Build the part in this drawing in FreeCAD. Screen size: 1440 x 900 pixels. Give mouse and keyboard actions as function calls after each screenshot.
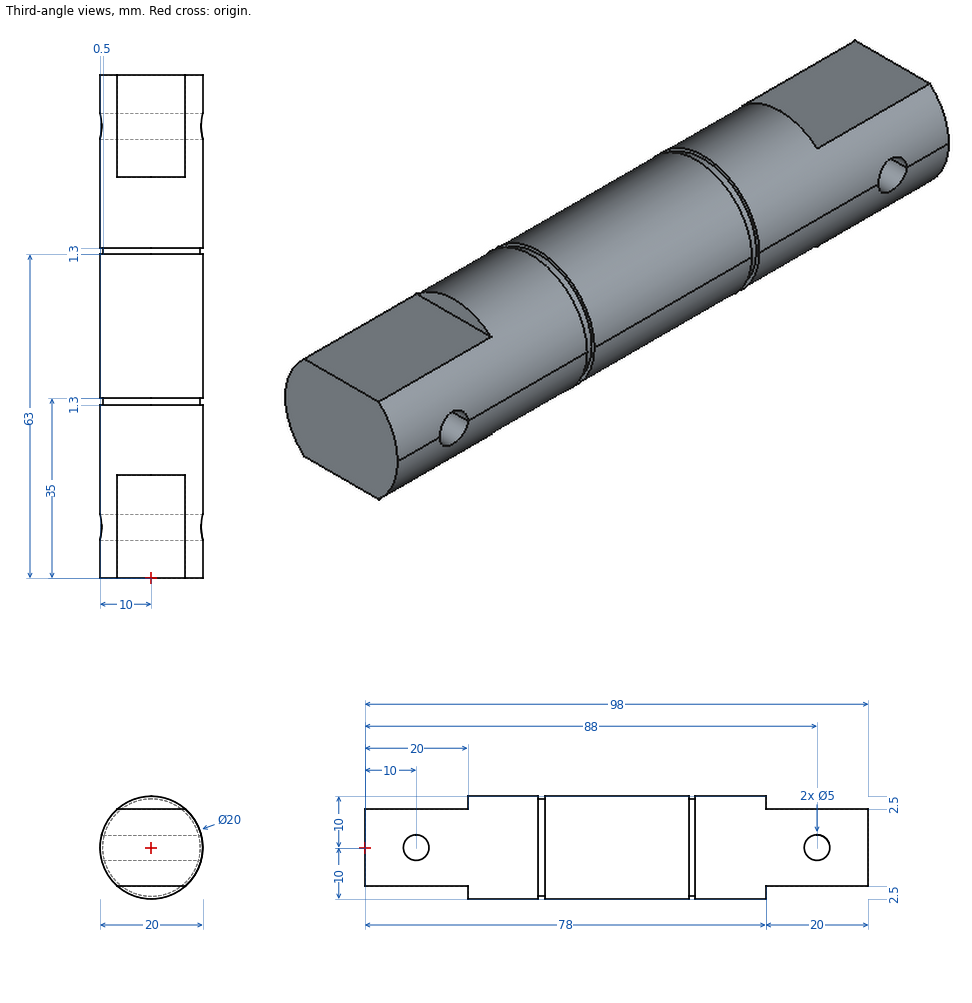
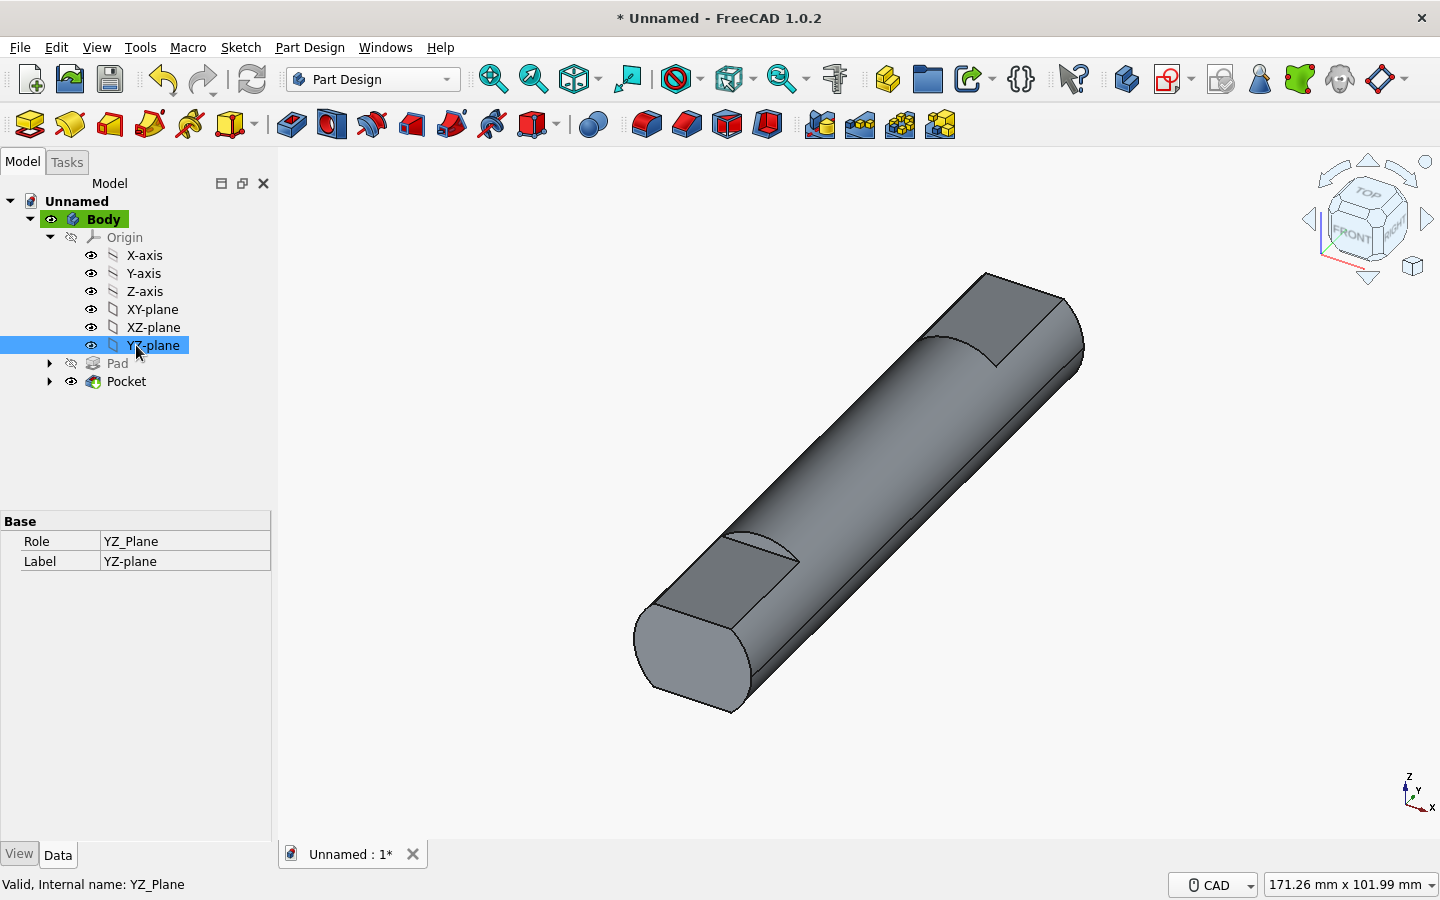
click(1380, 80)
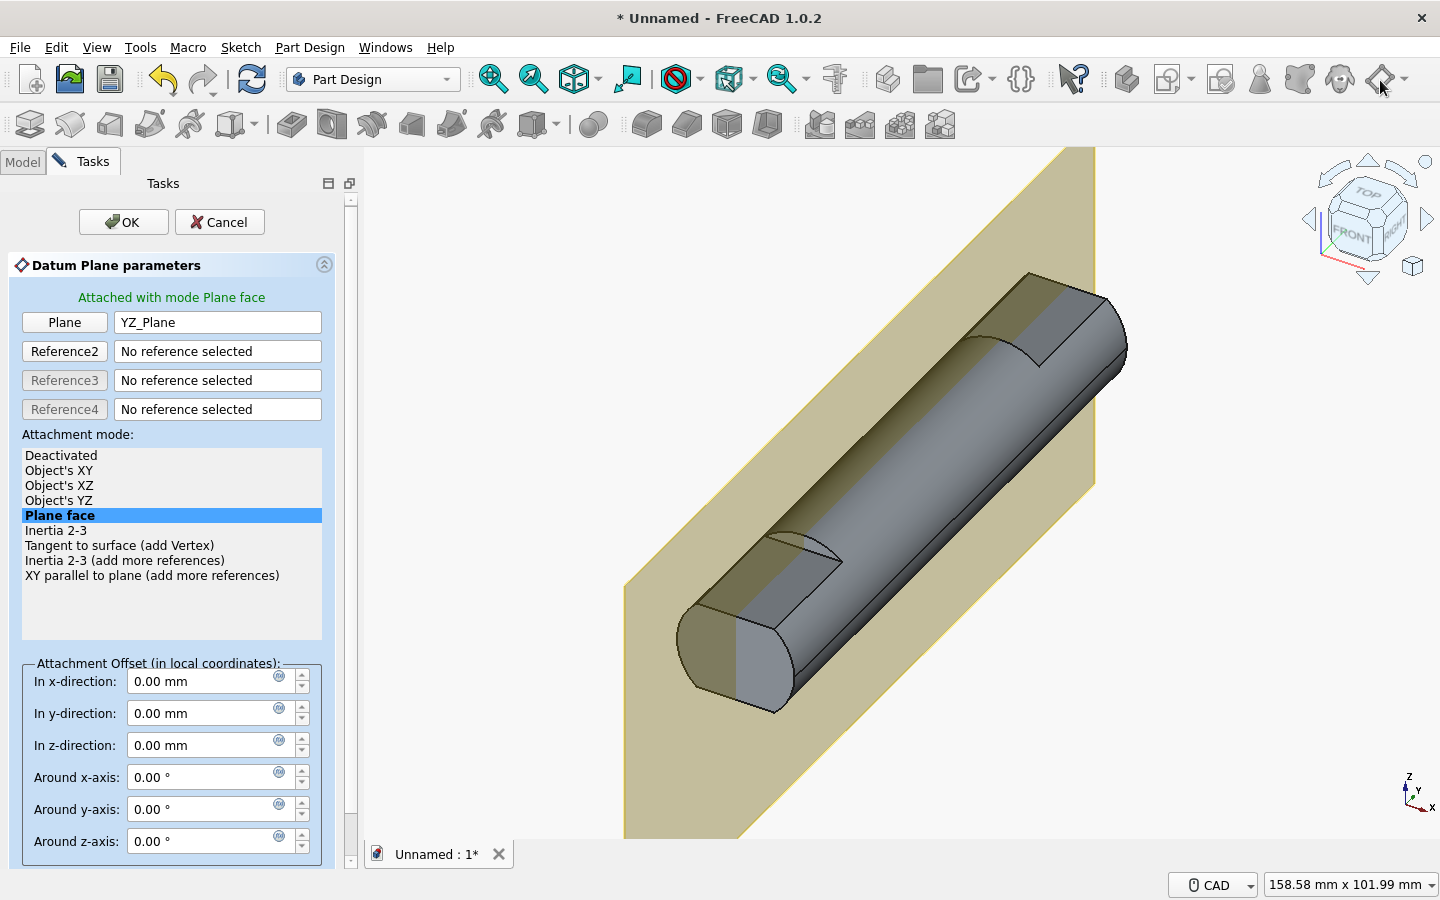
triple_click(210, 745)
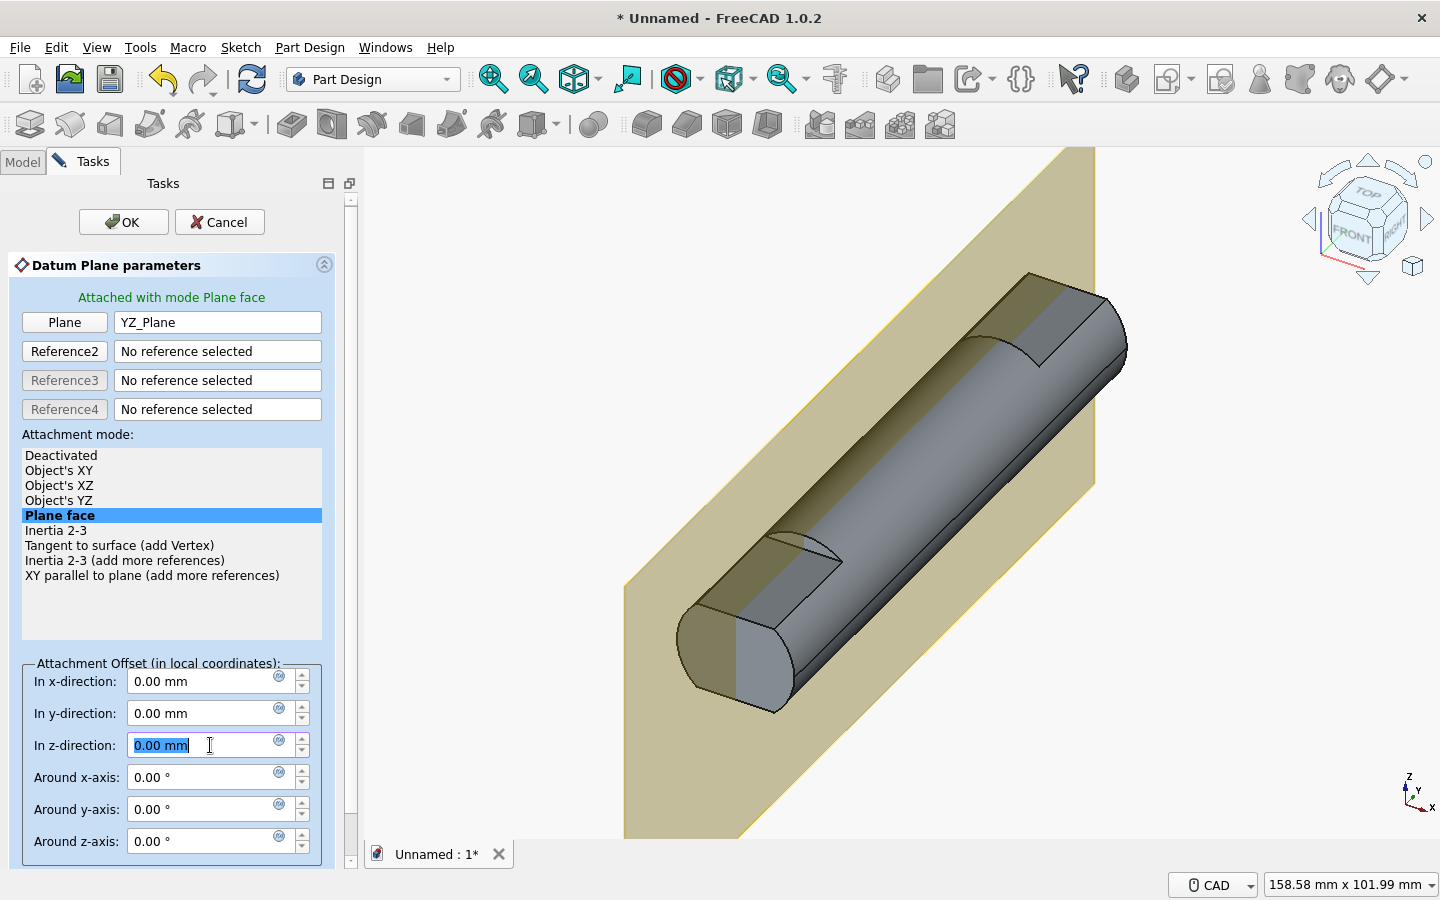
text(10)
key(Tab)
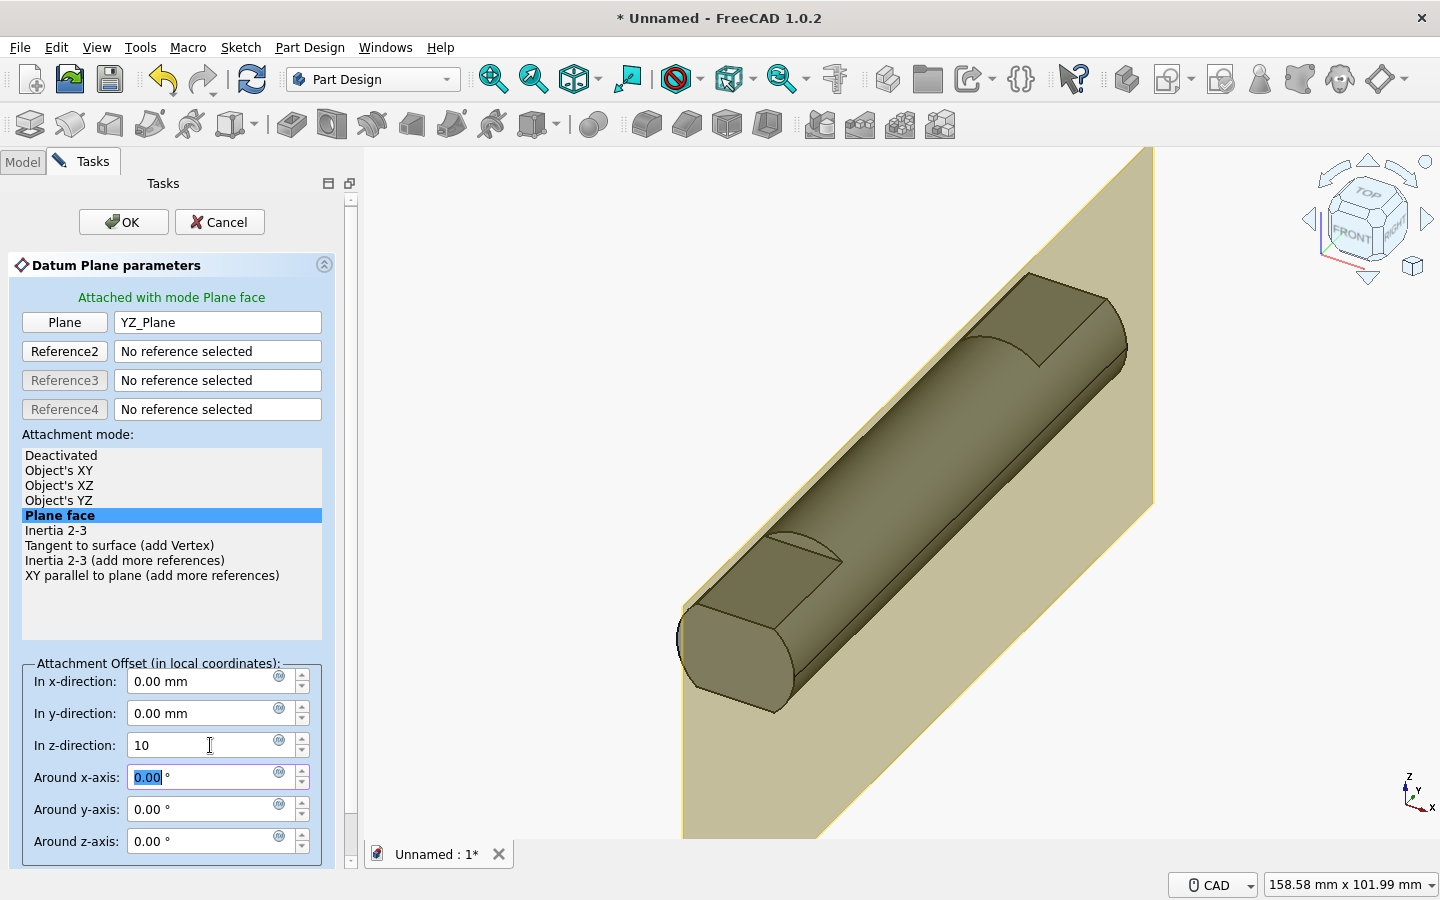
click(124, 222)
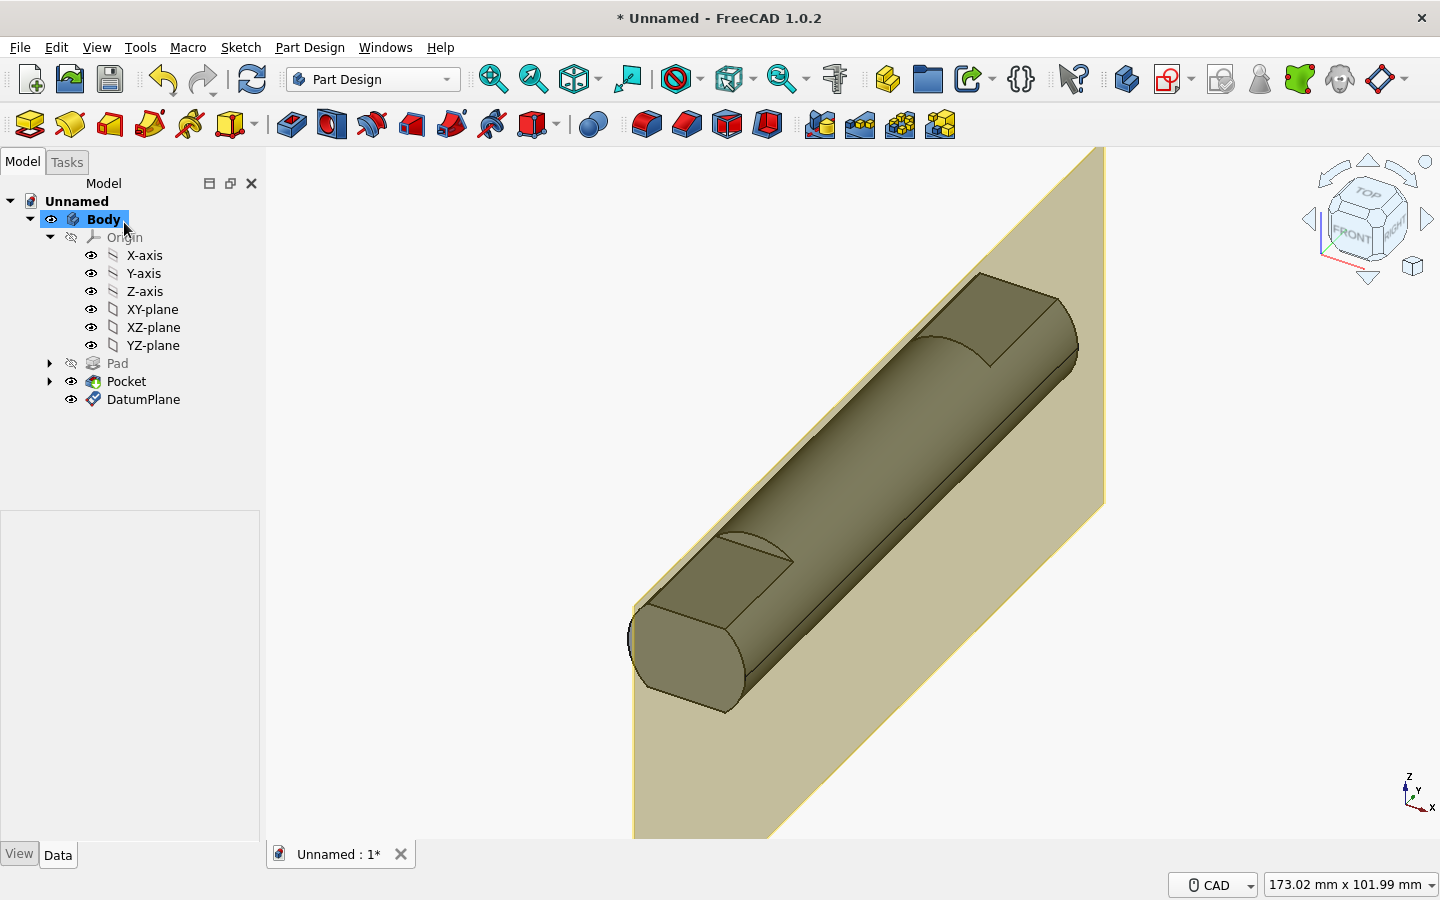
click(116, 399)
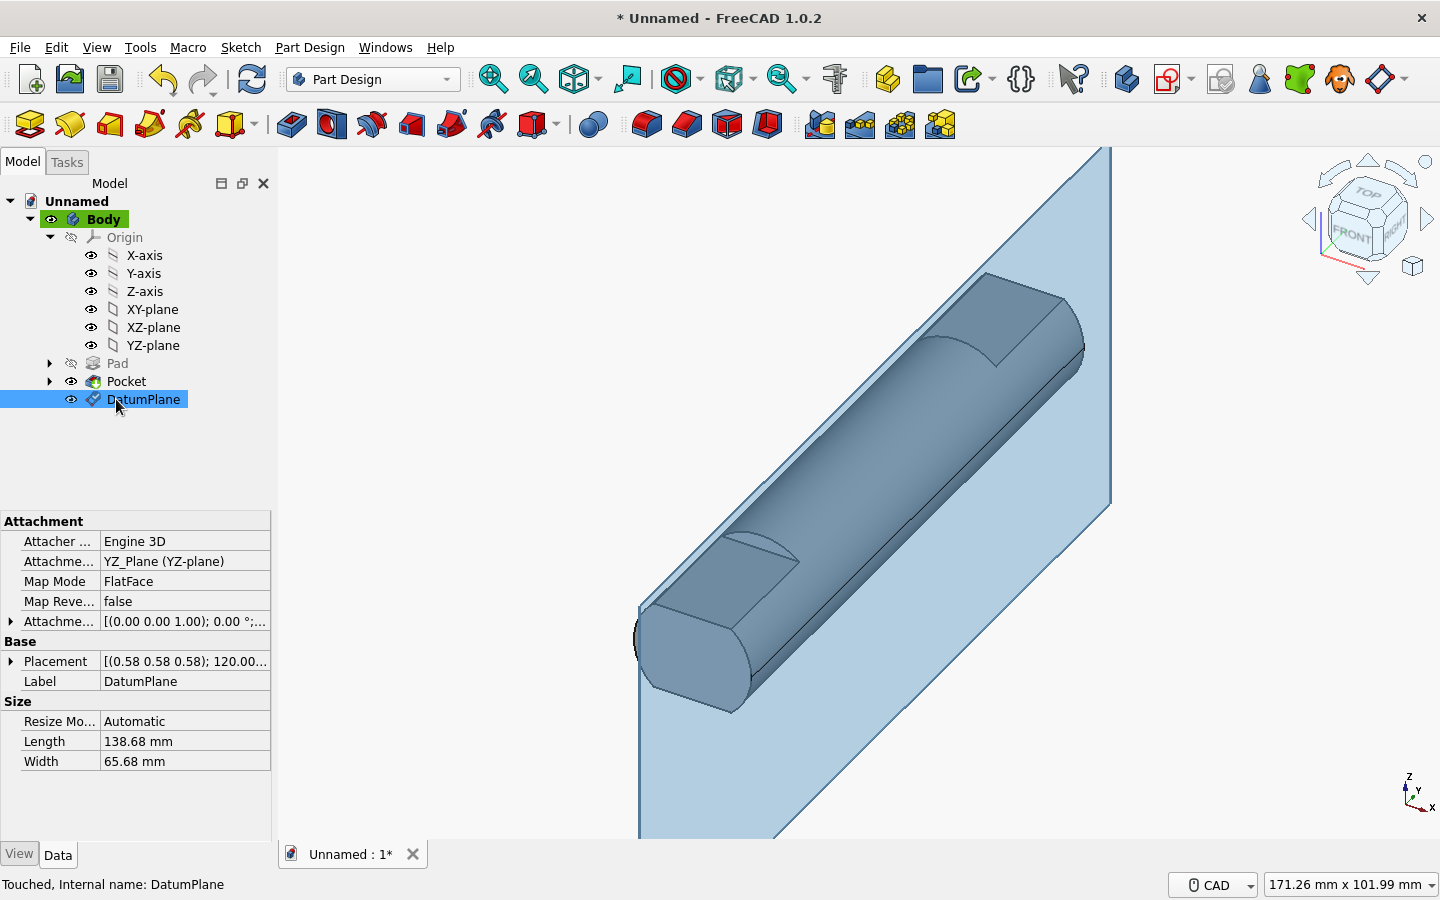
click(1168, 80)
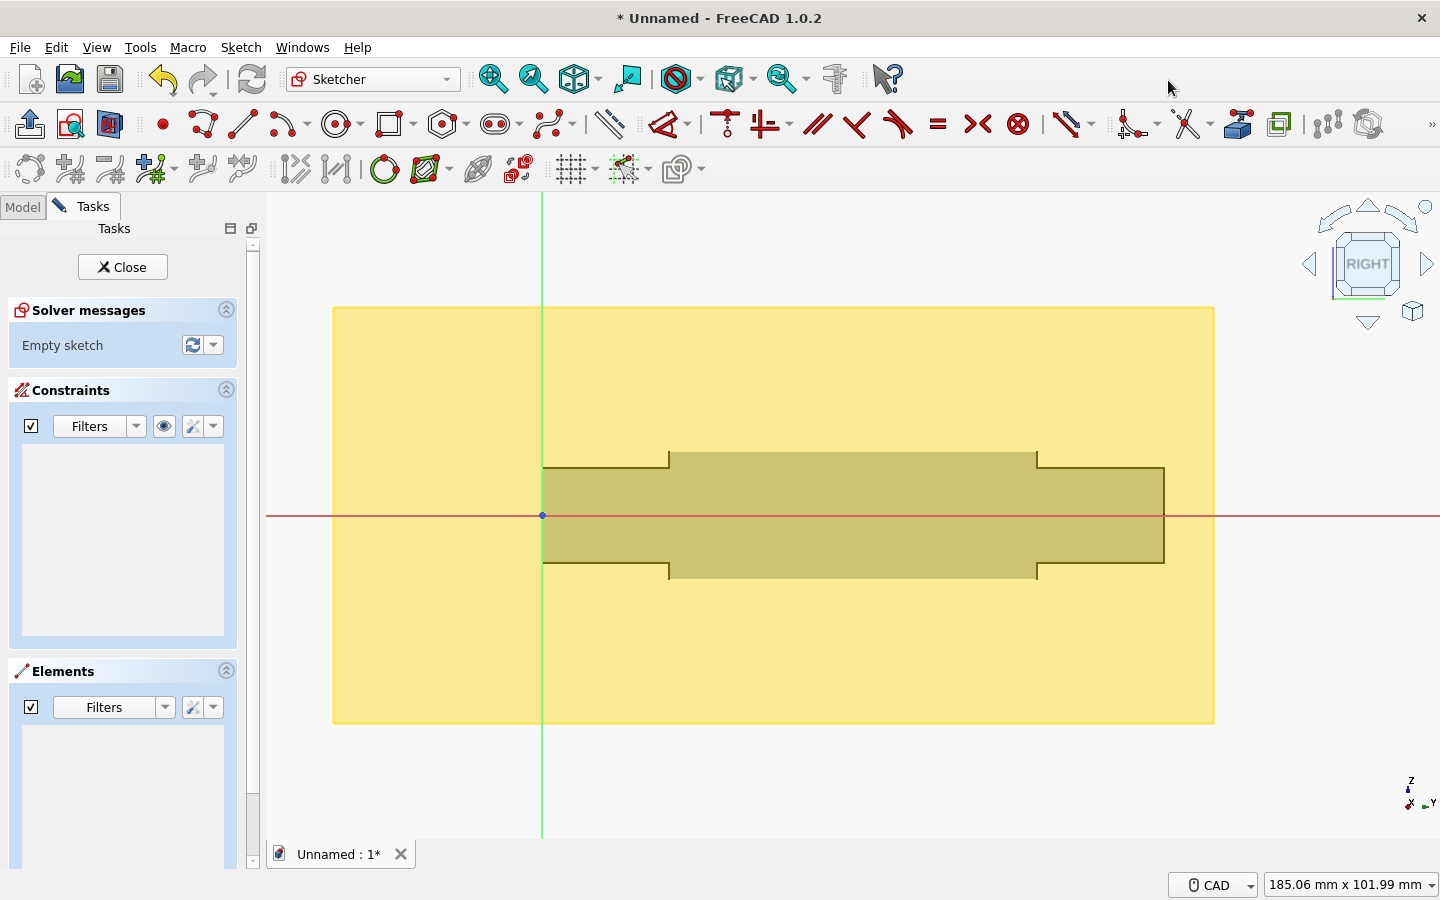
click(336, 124)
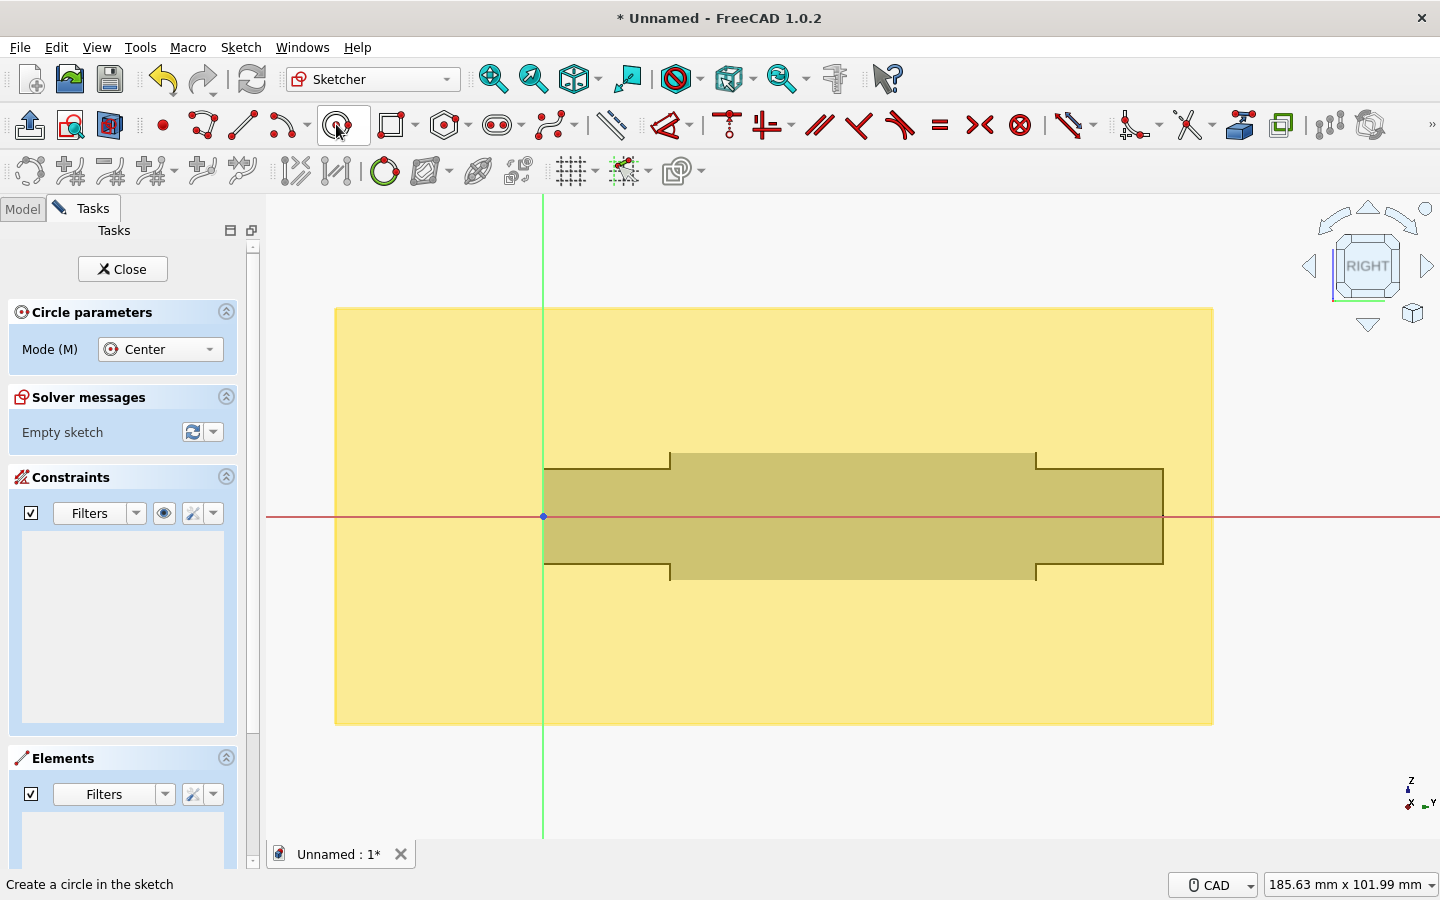
scroll(1100, 517, up, 2)